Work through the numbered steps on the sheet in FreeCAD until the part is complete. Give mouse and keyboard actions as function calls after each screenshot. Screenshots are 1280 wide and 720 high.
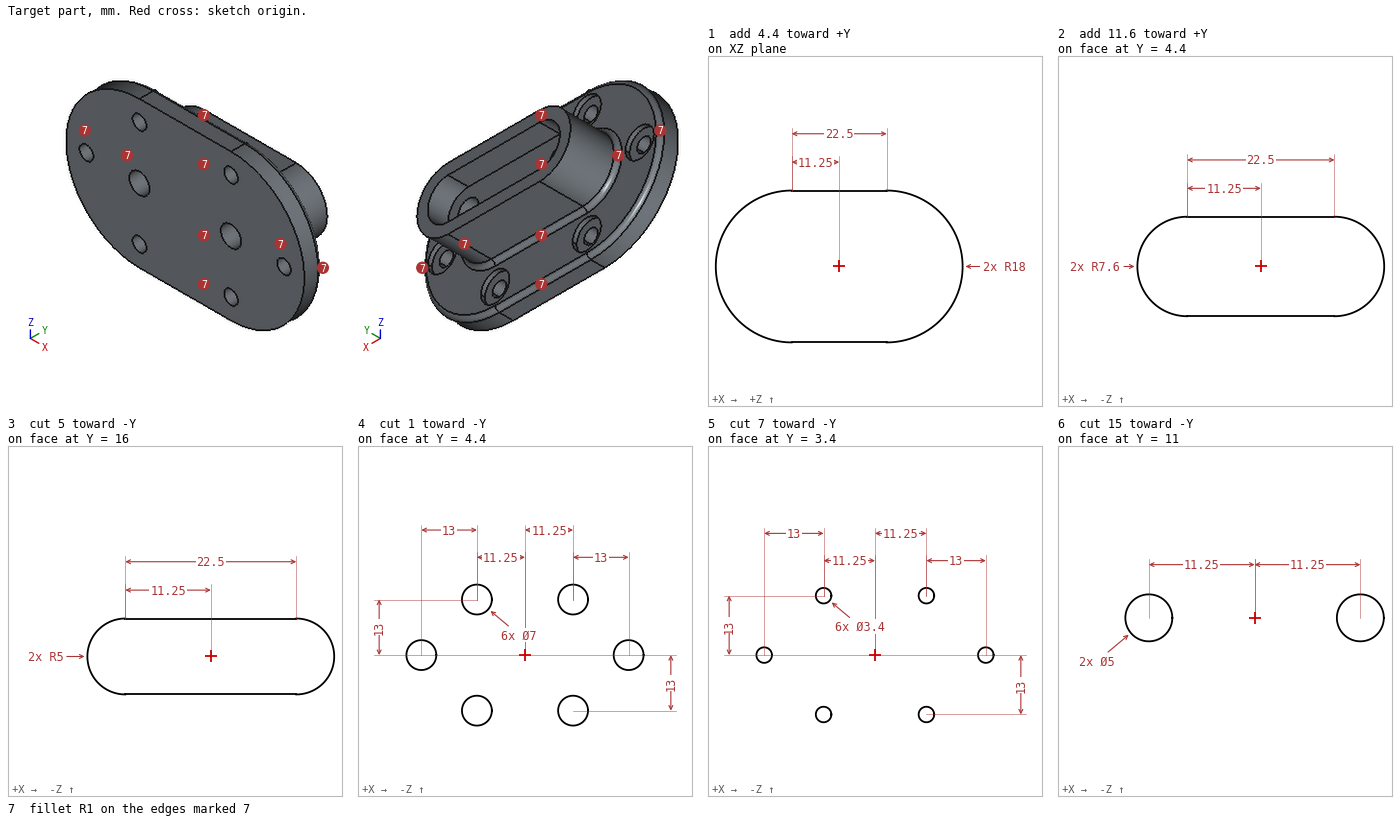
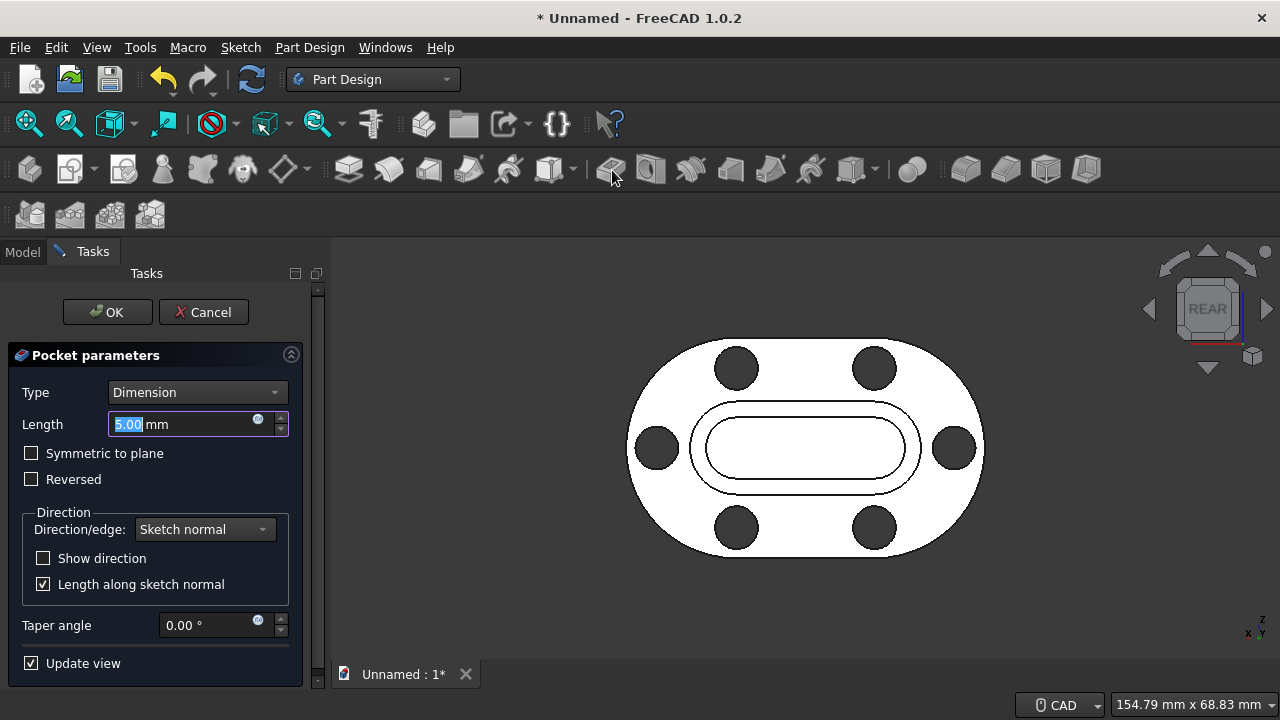
text(1)
key(Tab)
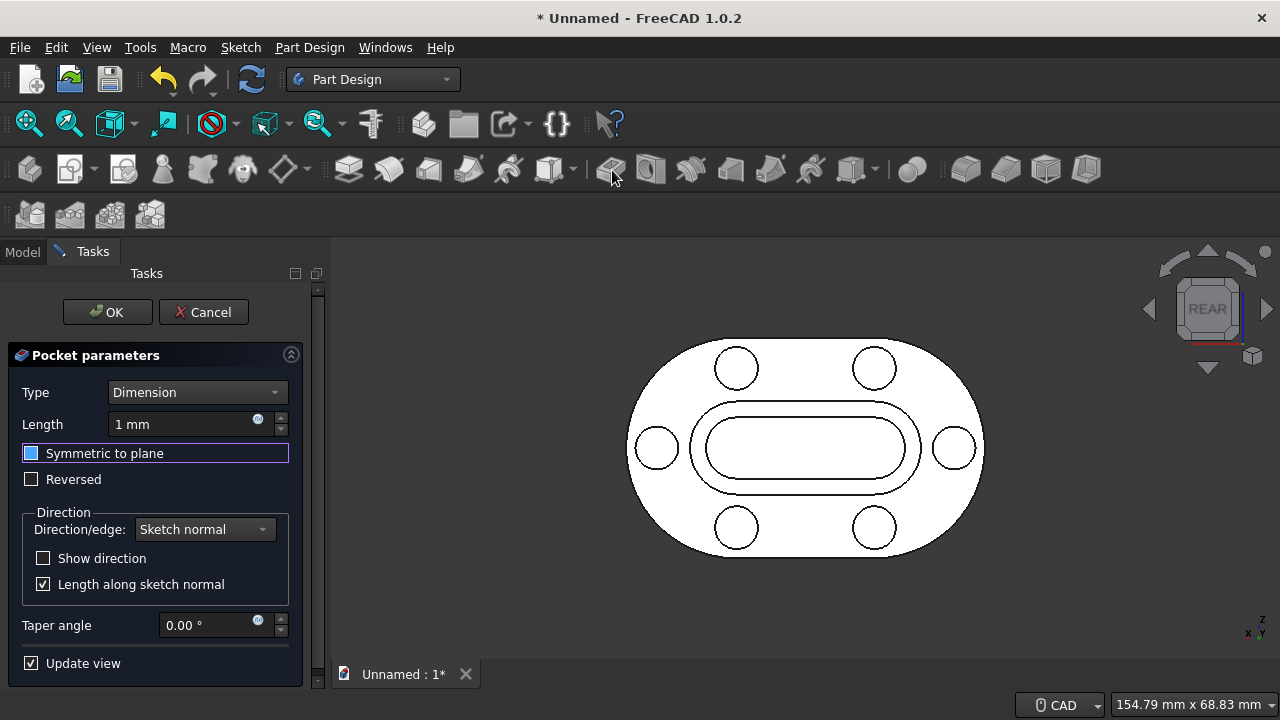
click(108, 312)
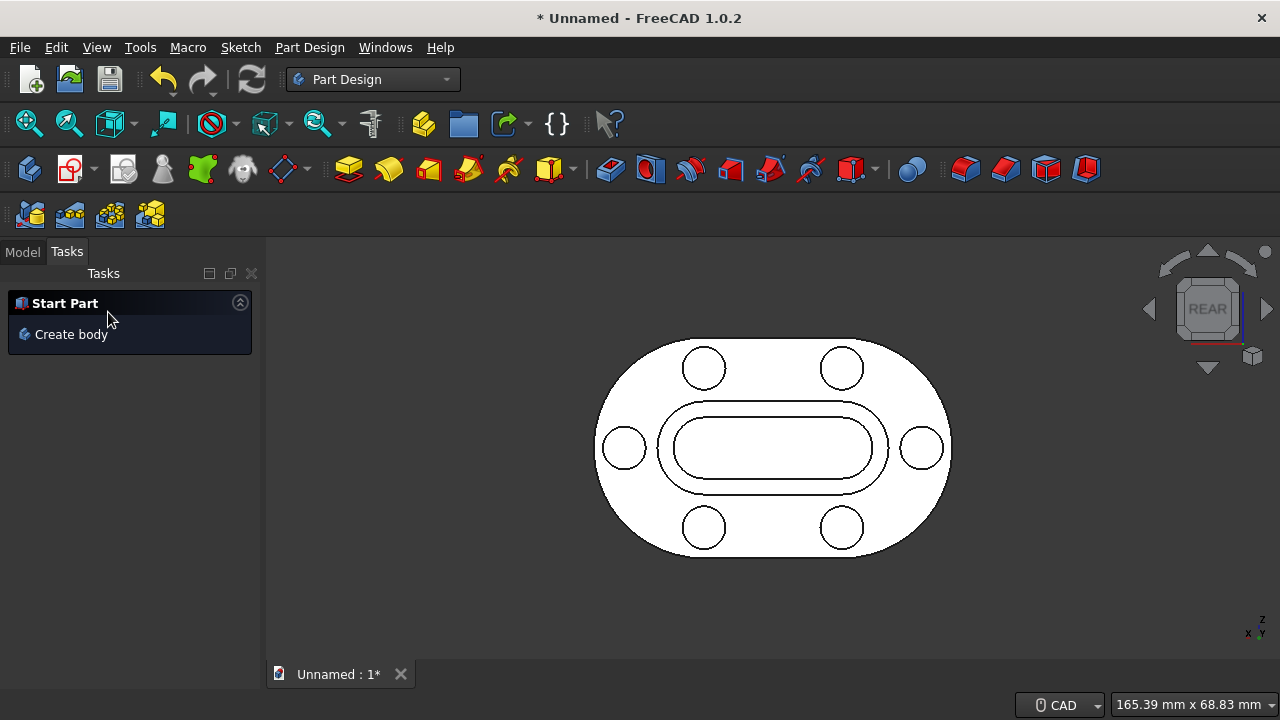
click(624, 447)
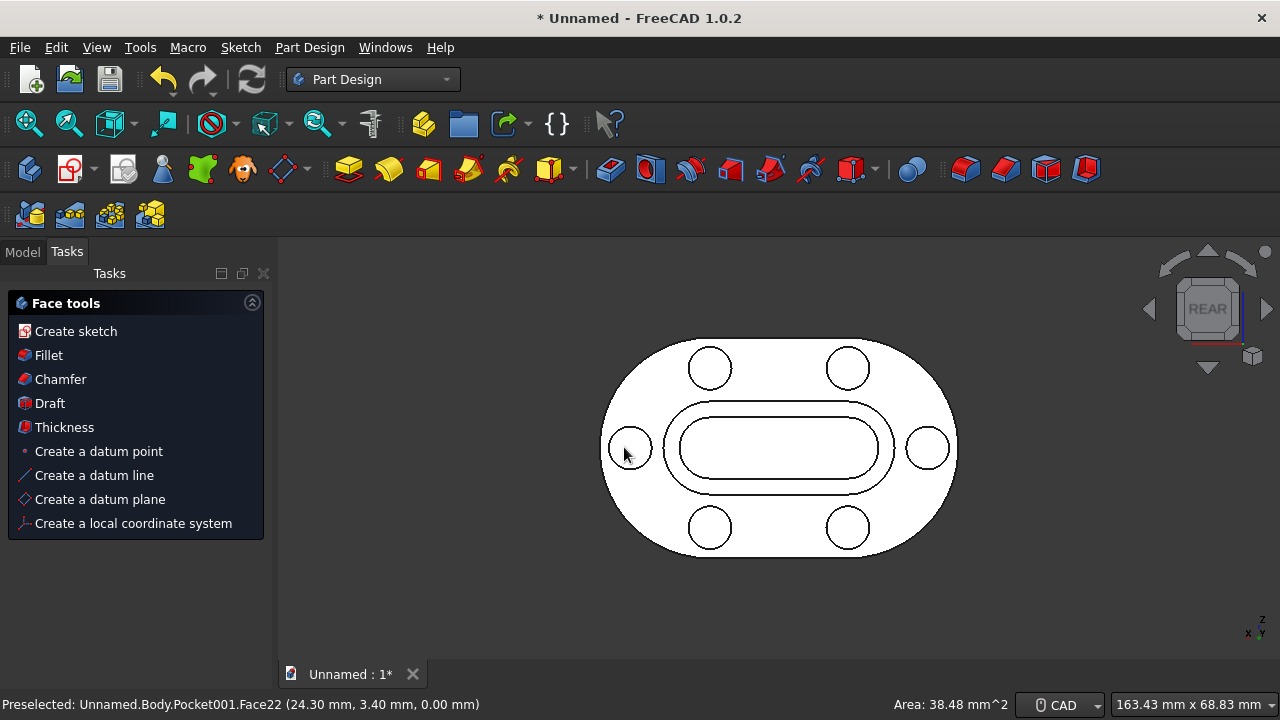
click(70, 170)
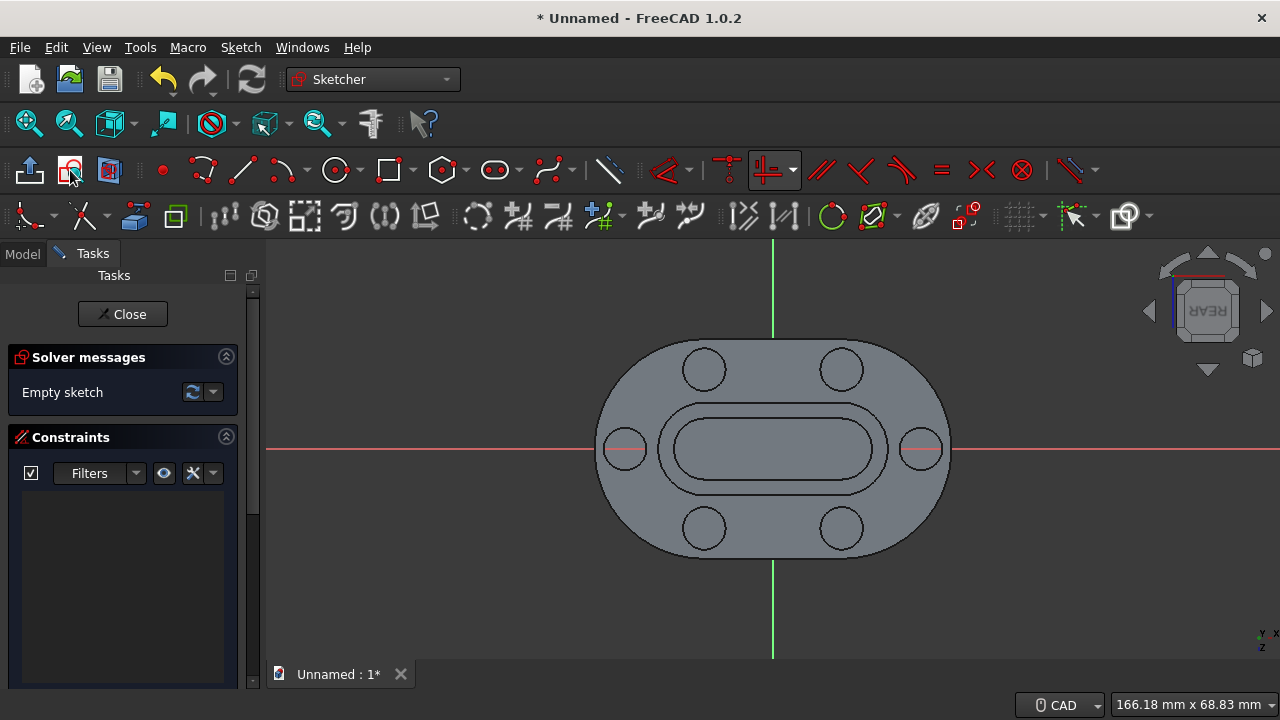
click(110, 170)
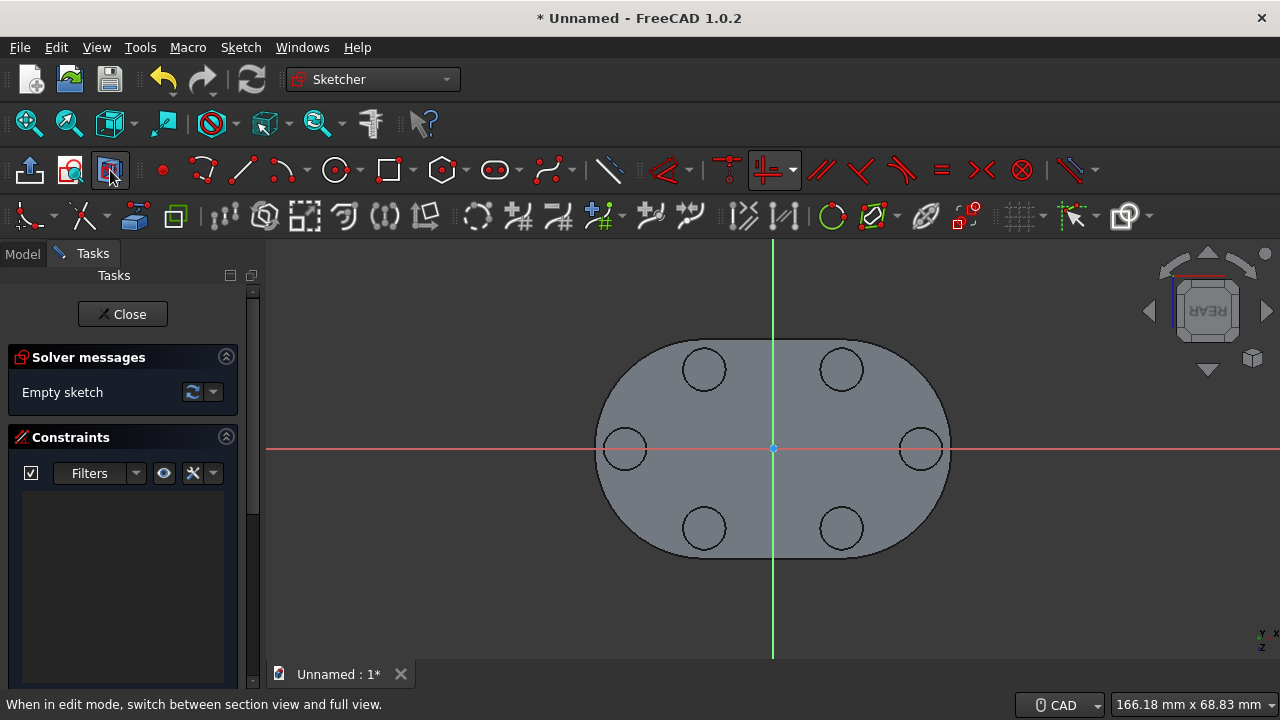
scroll(912, 449, up, 2)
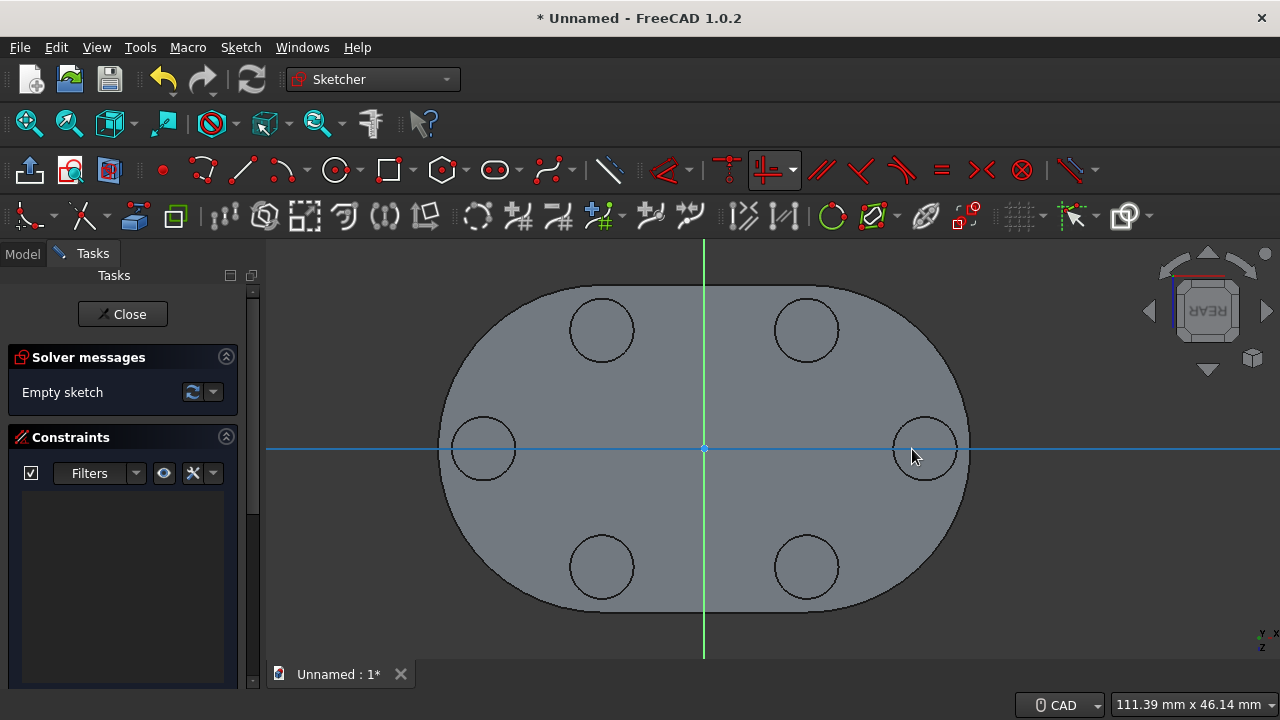
click(336, 170)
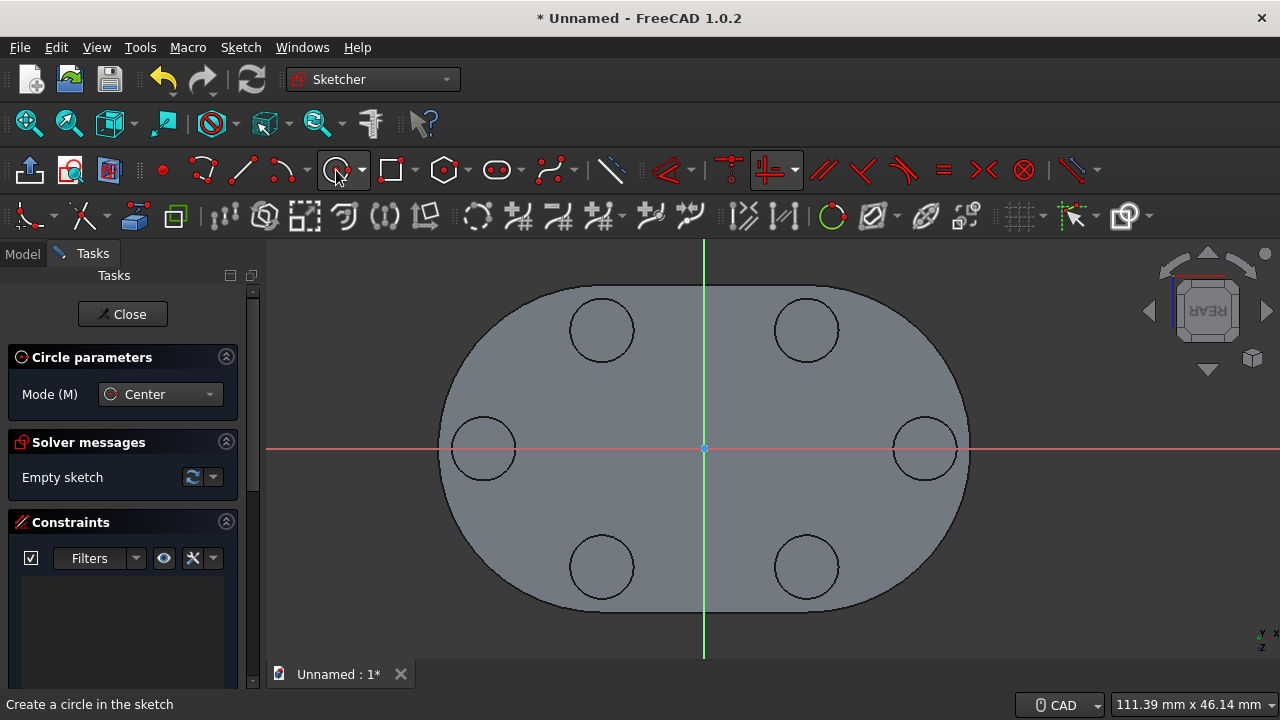
scroll(602, 330, up, 2)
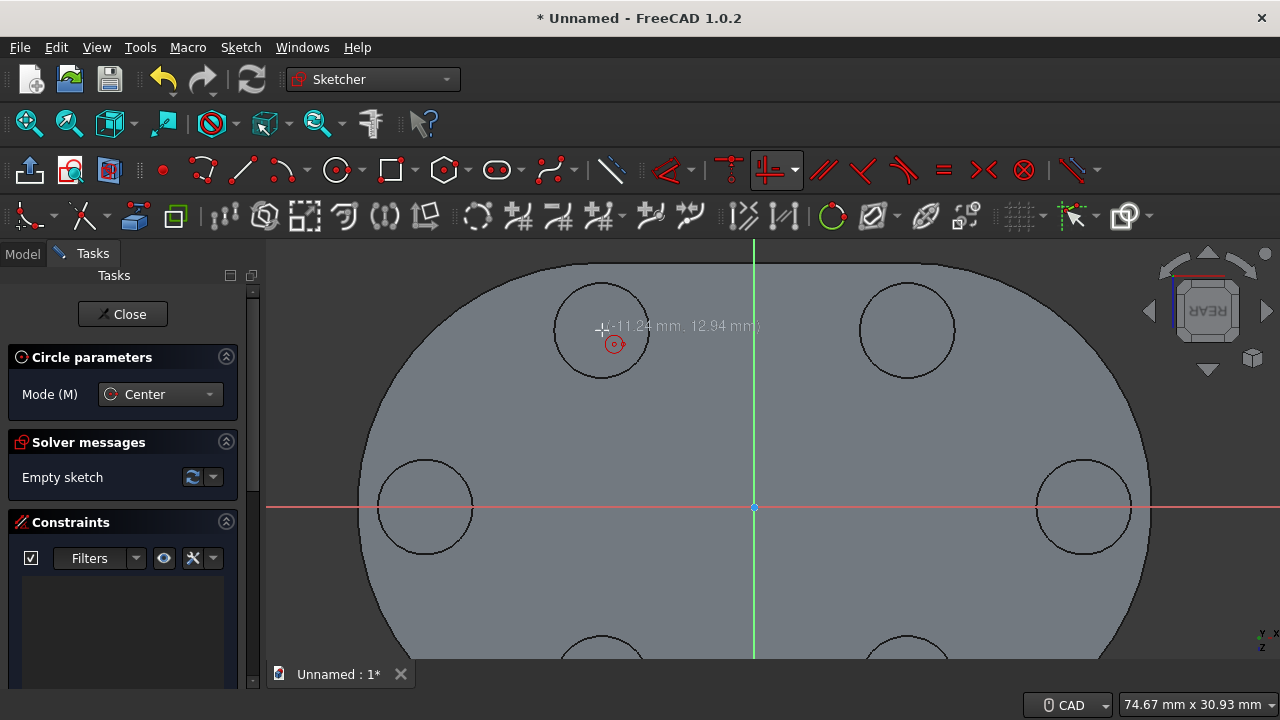
click(602, 331)
move(618, 314)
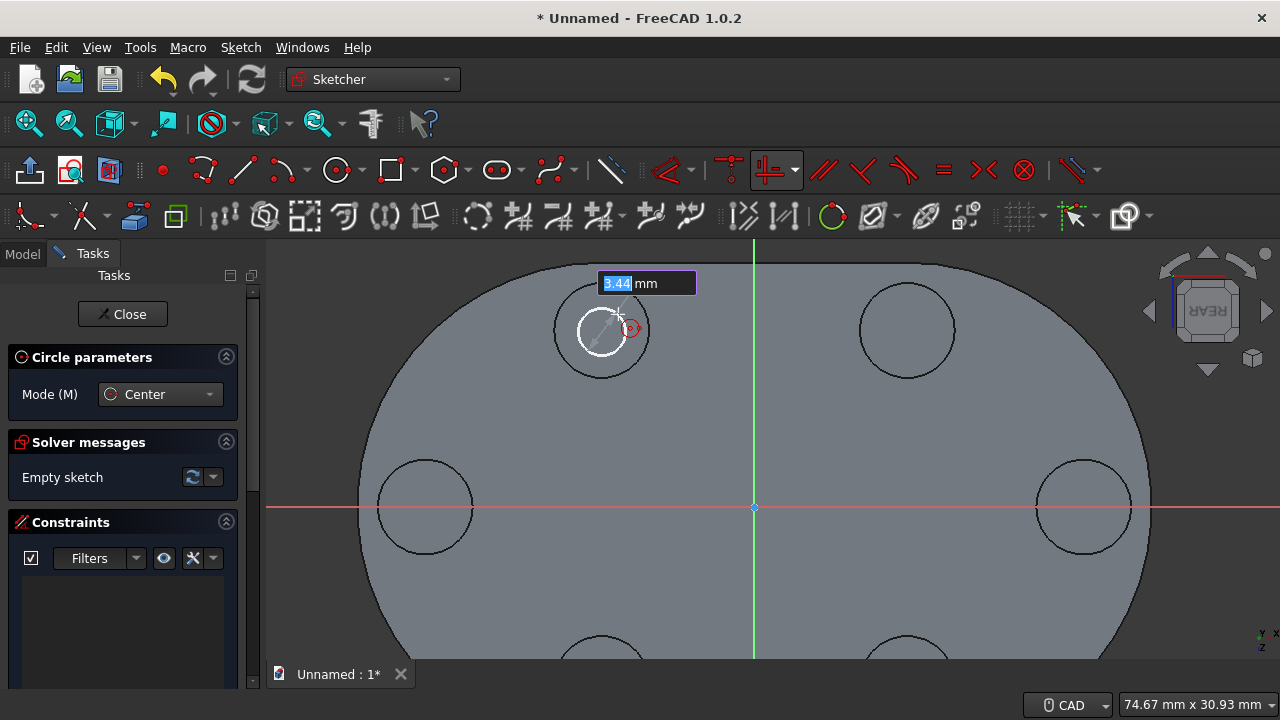
text(3.4)
key(Return)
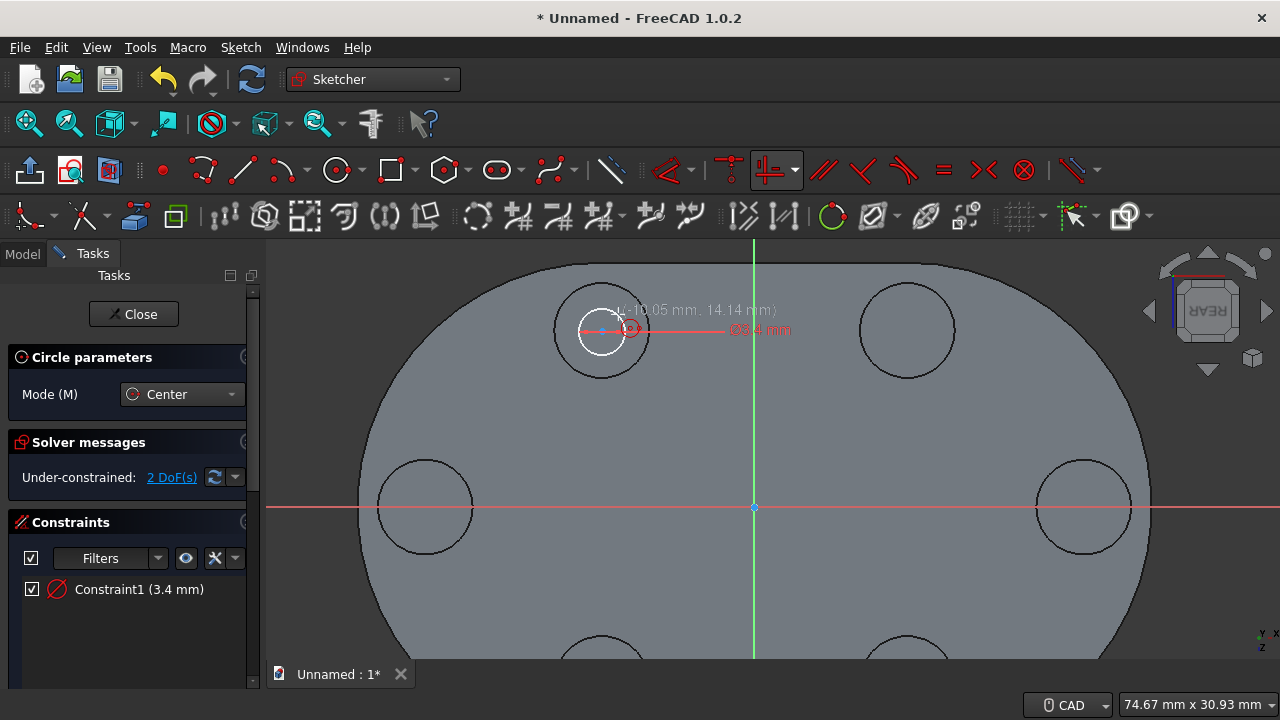
click(907, 331)
move(924, 314)